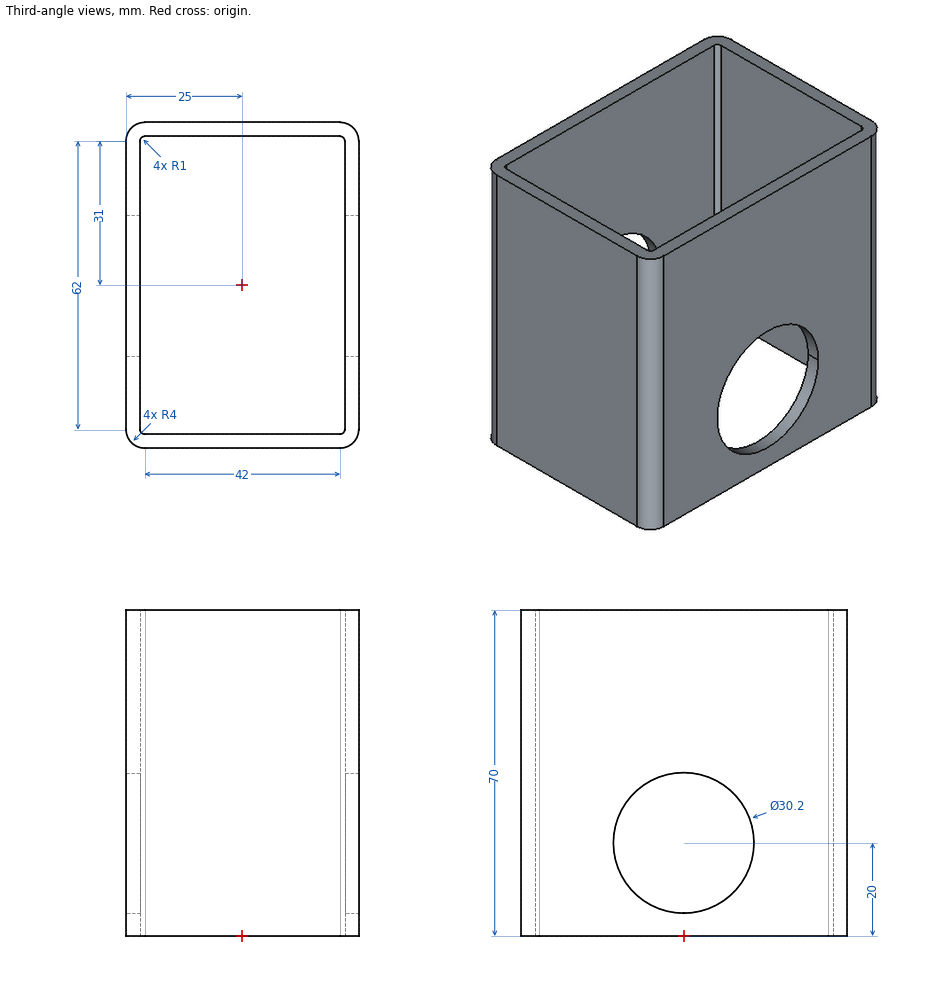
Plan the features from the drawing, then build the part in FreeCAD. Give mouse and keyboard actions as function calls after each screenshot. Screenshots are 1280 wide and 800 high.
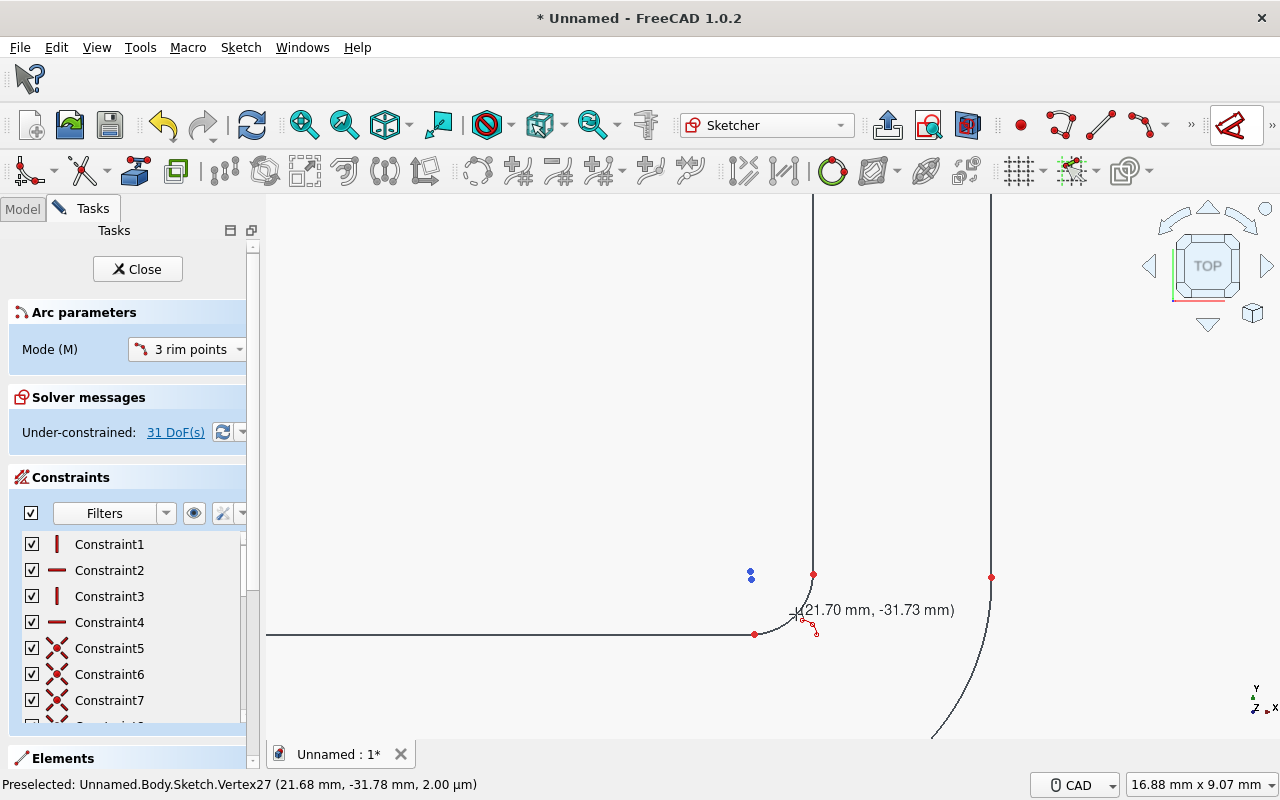
scroll(802, 608, down, 13)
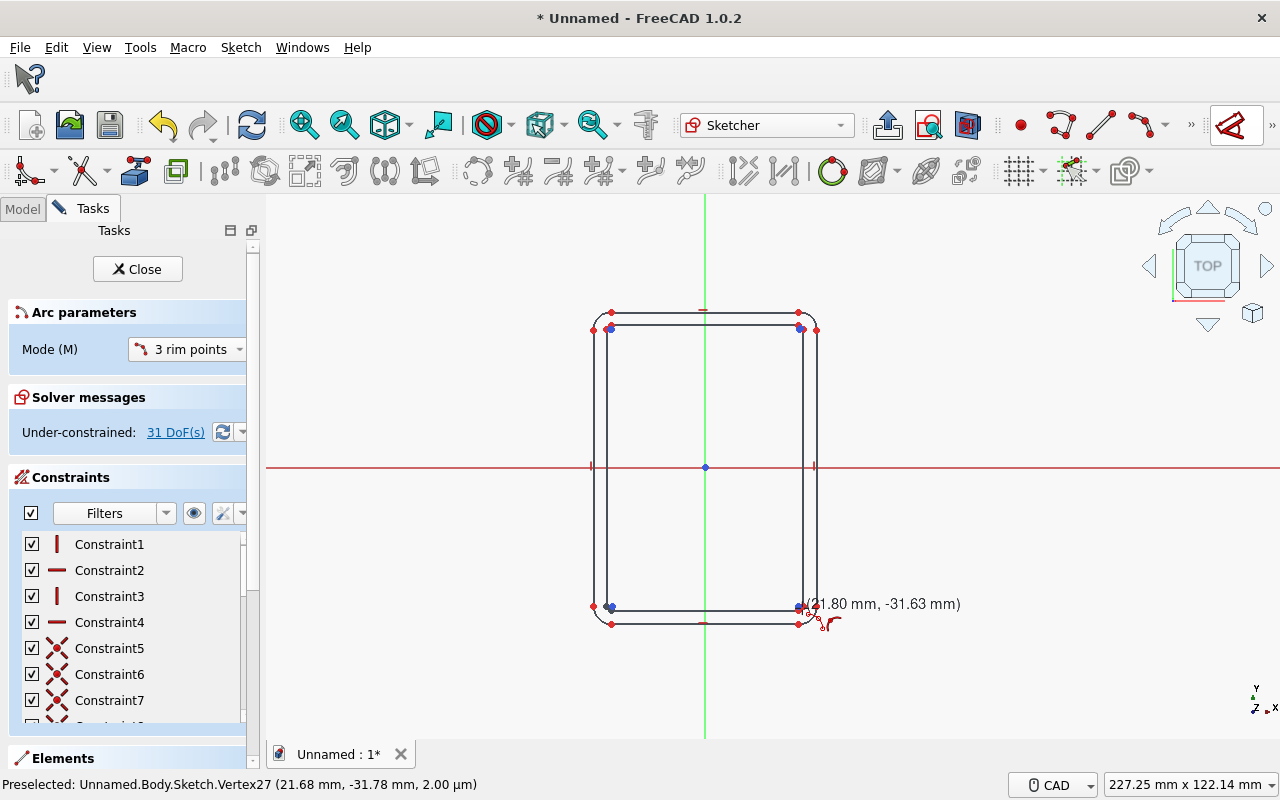
scroll(612, 610, up, 7)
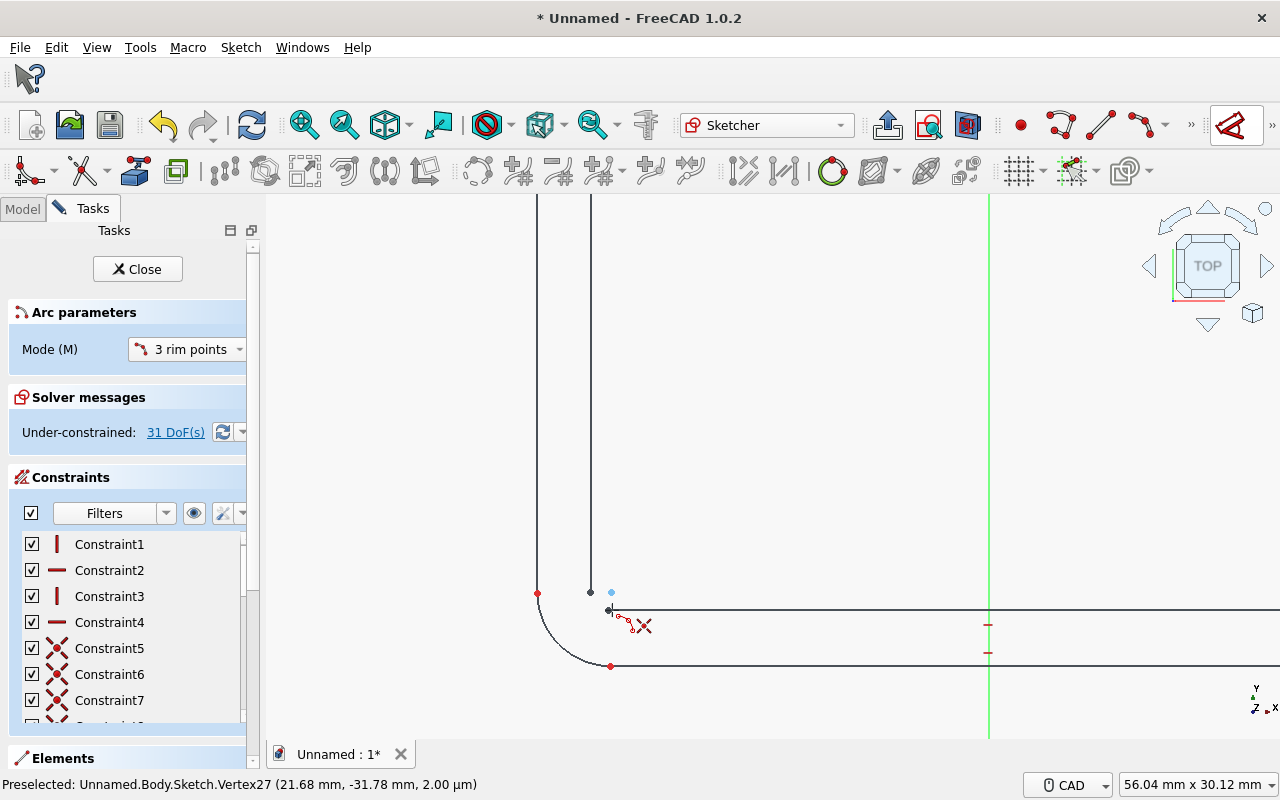
click(609, 610)
click(591, 592)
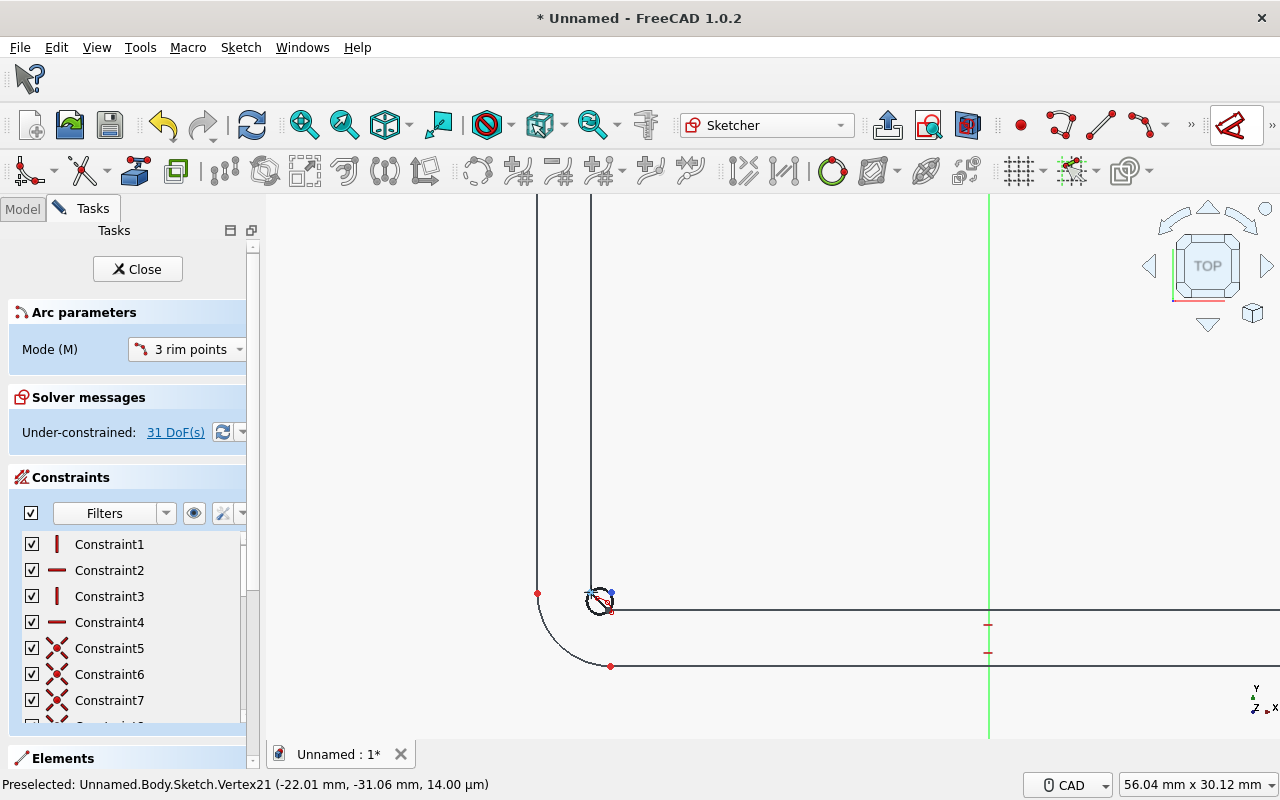
scroll(596, 604, up, 6)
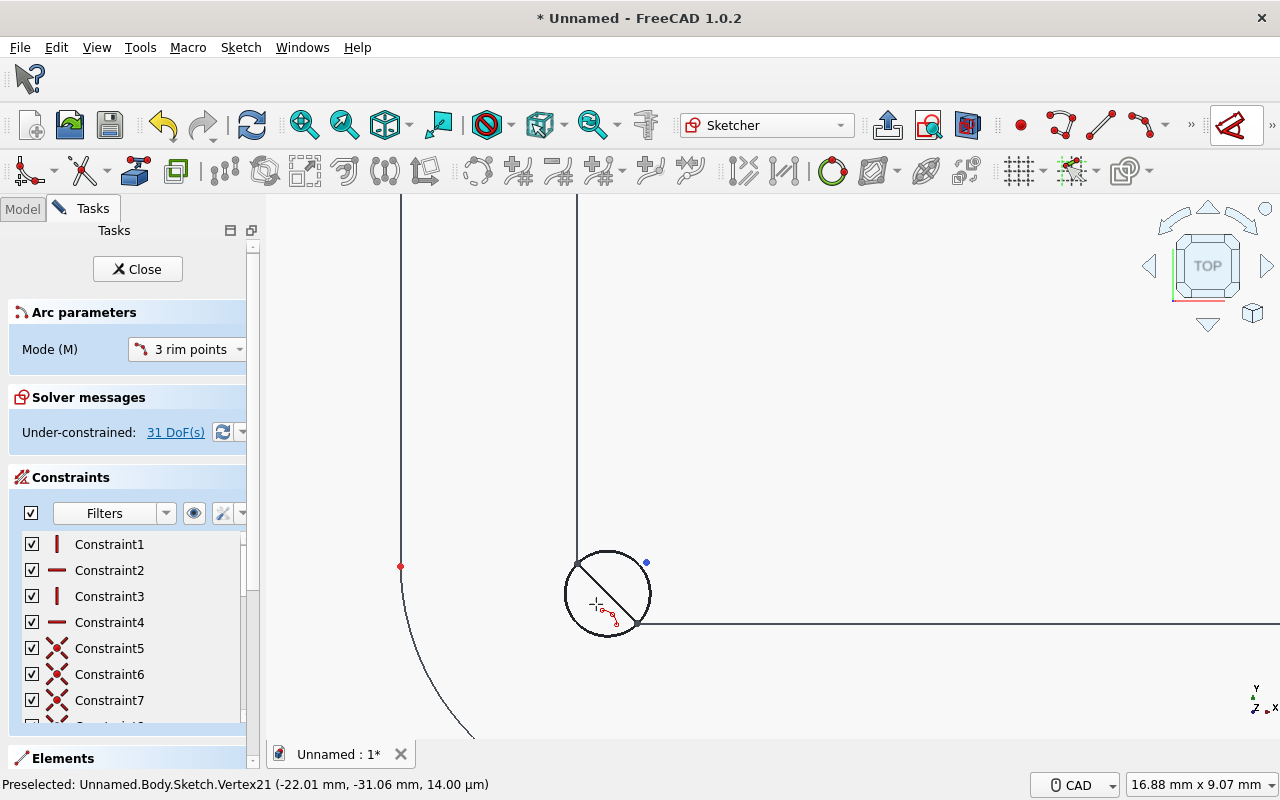
click(596, 603)
key(Escape)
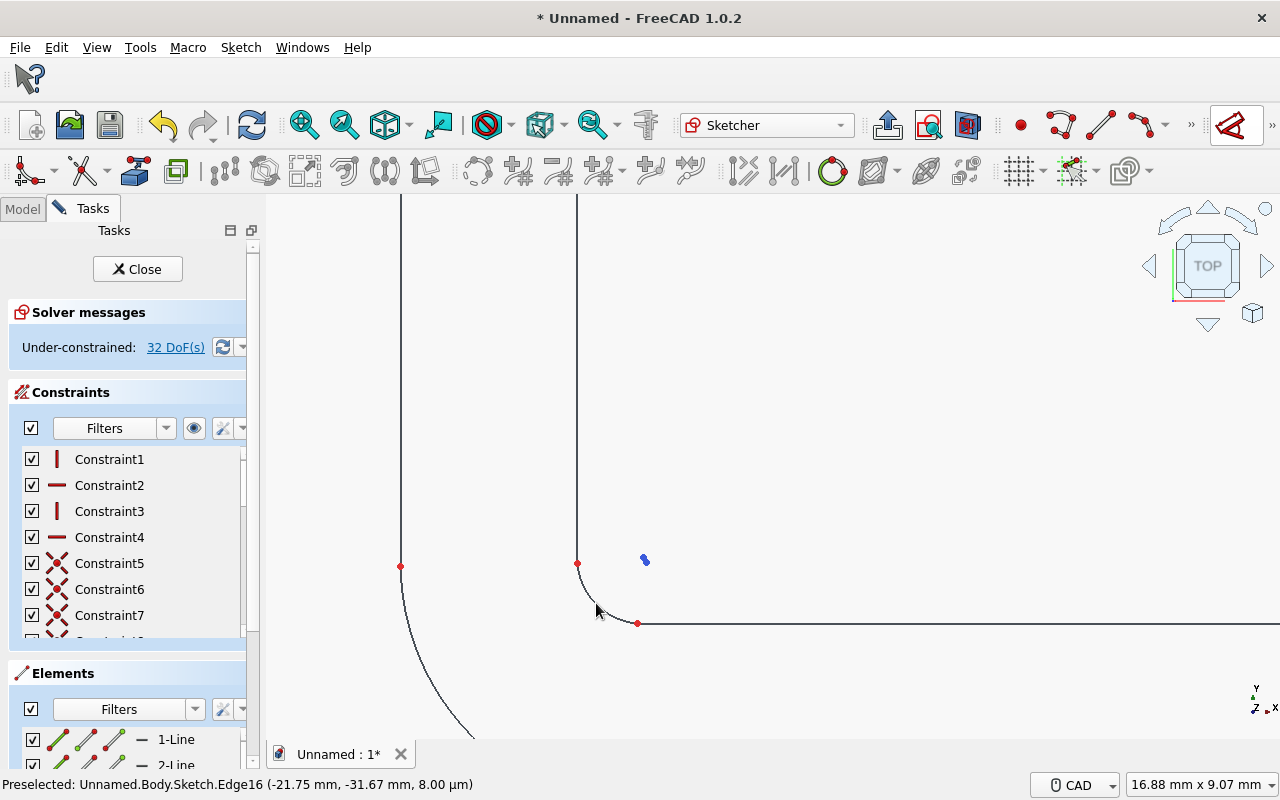
scroll(609, 608, down, 13)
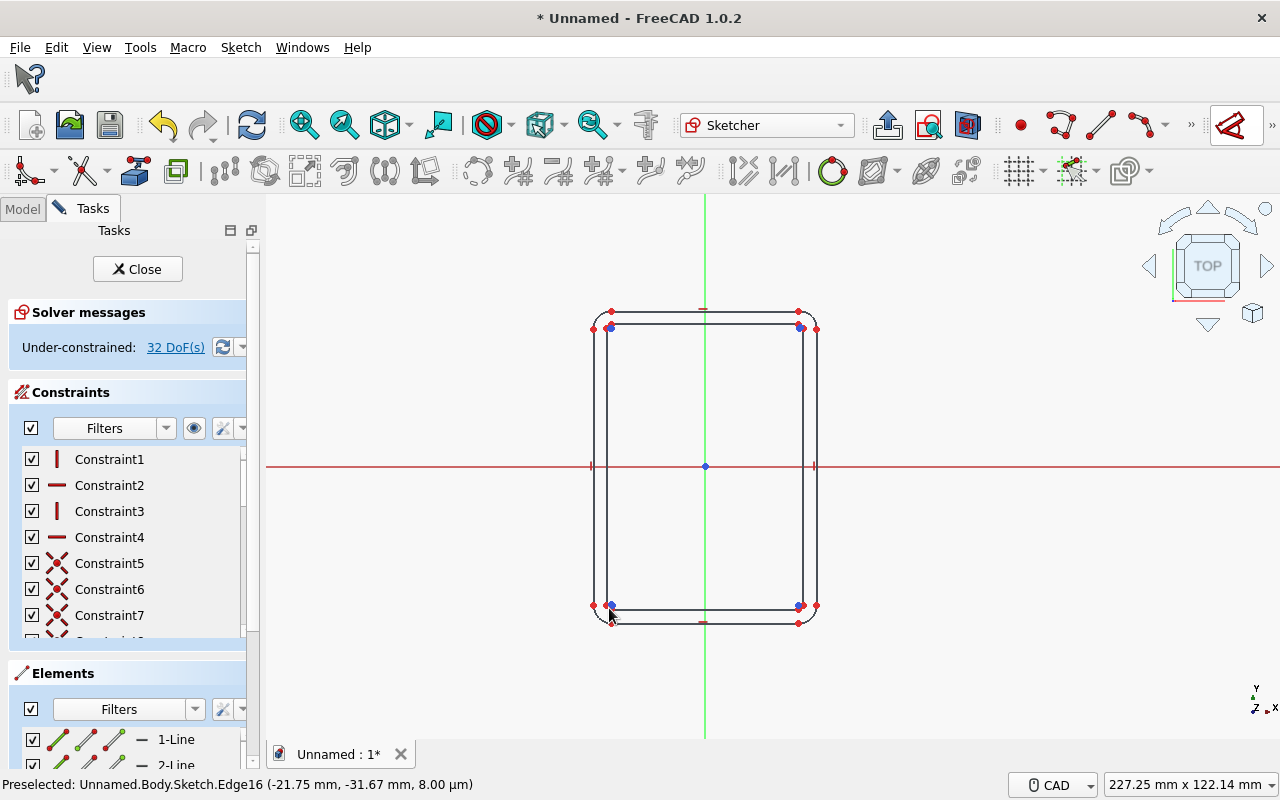
click(594, 412)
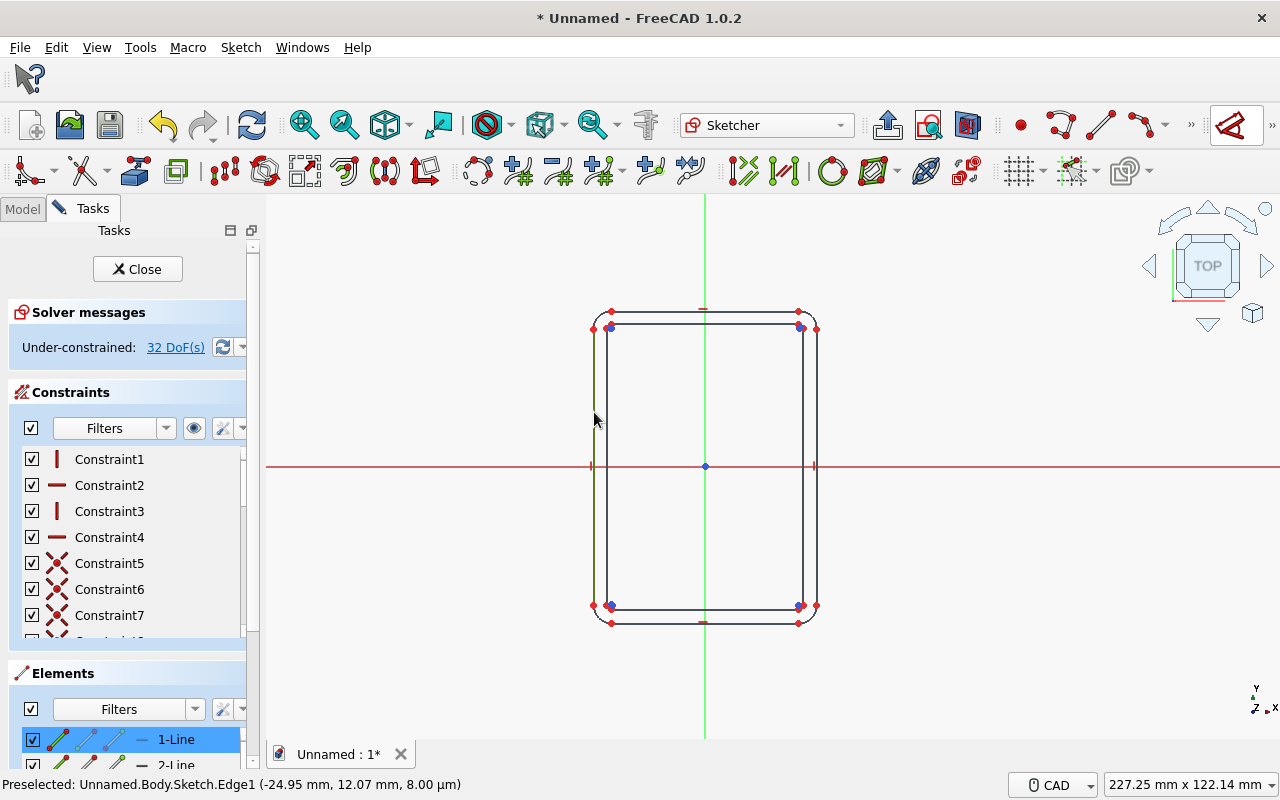
click(599, 618)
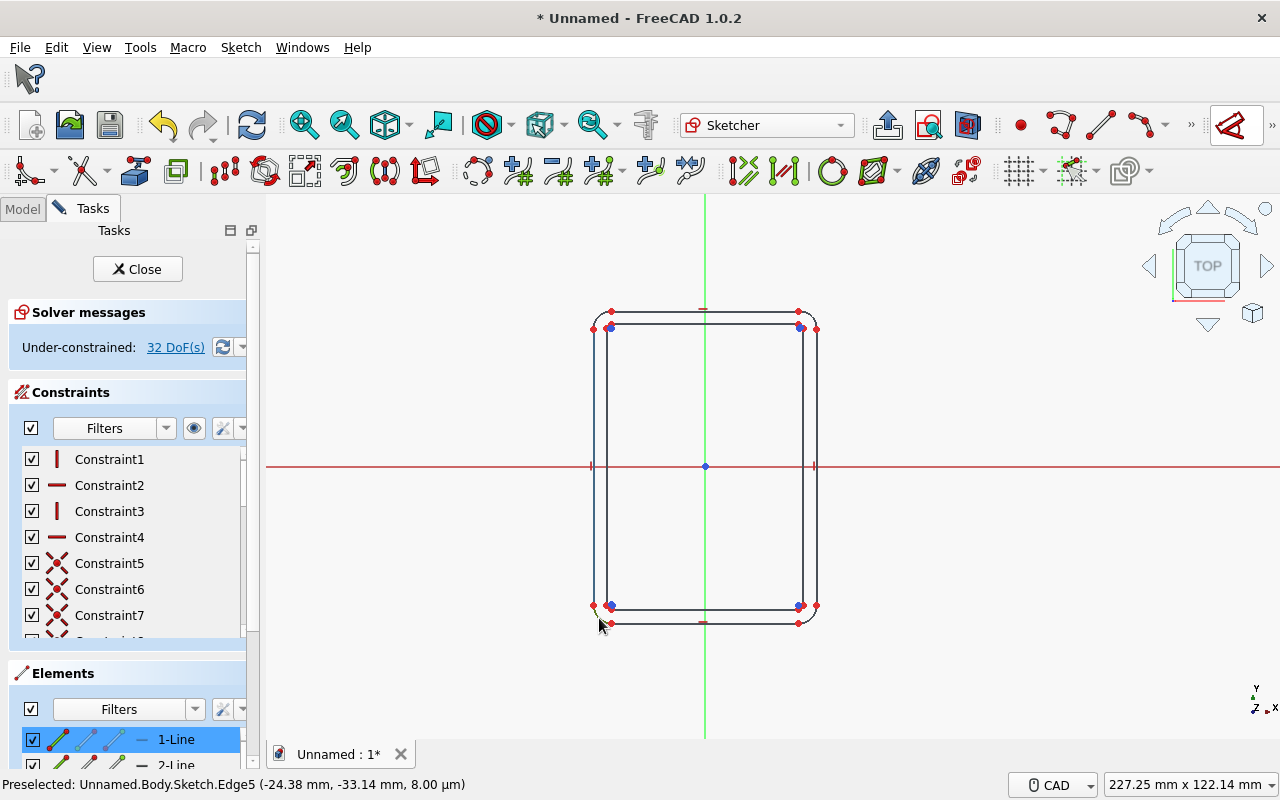
key(t)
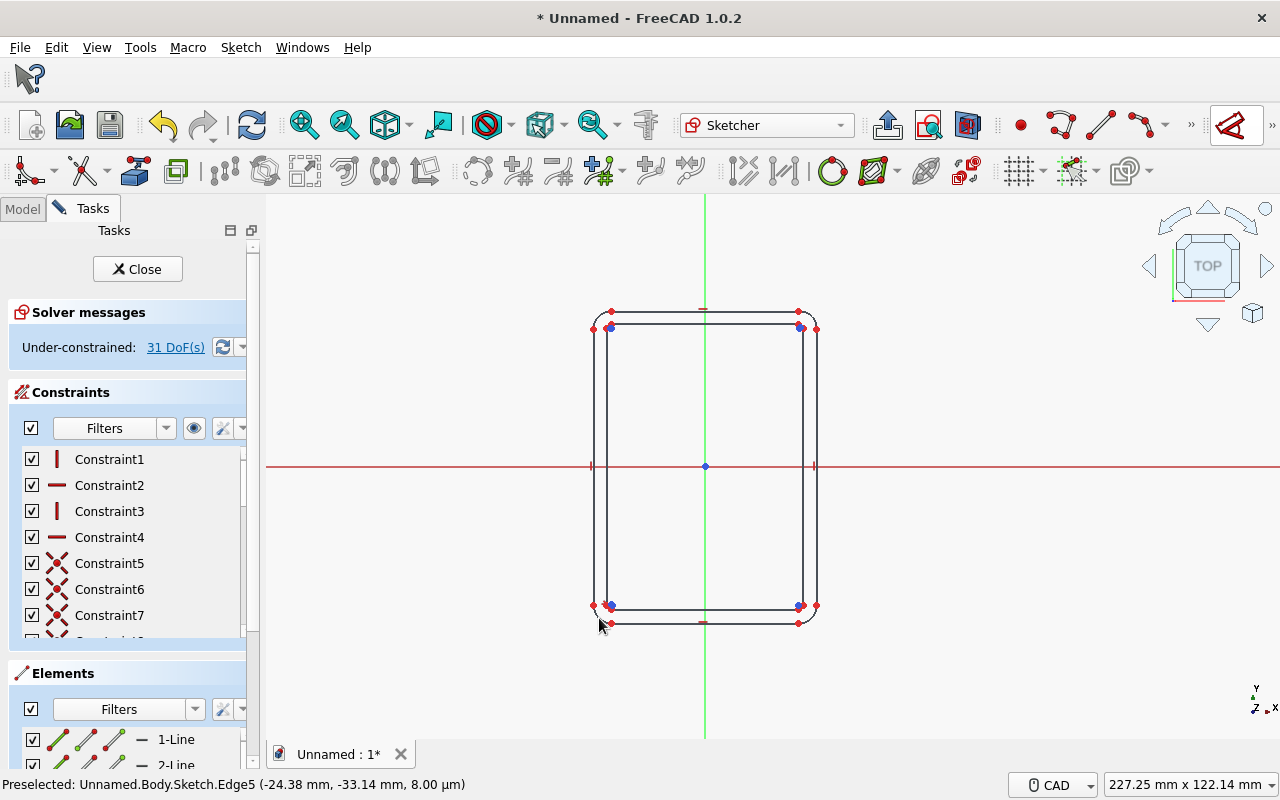
click(594, 412)